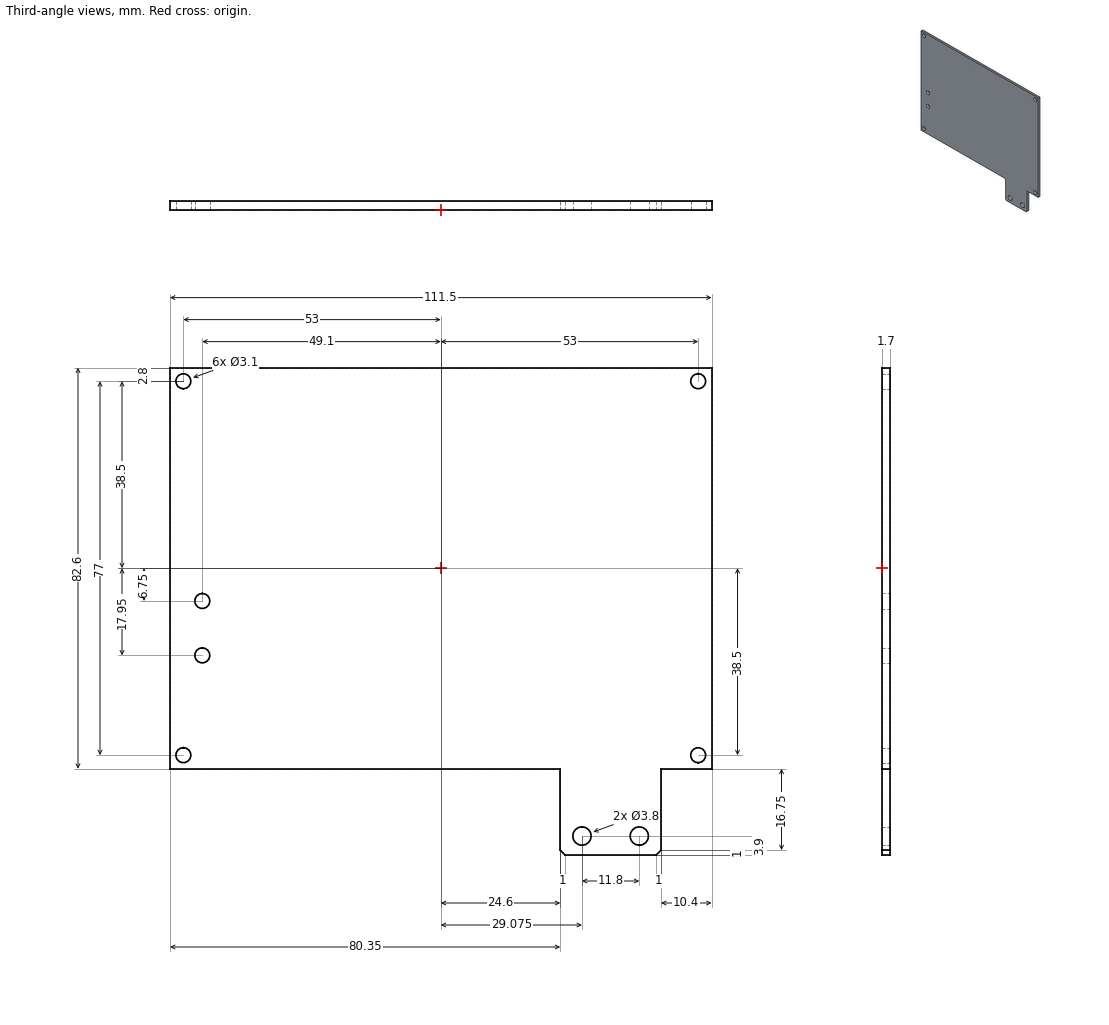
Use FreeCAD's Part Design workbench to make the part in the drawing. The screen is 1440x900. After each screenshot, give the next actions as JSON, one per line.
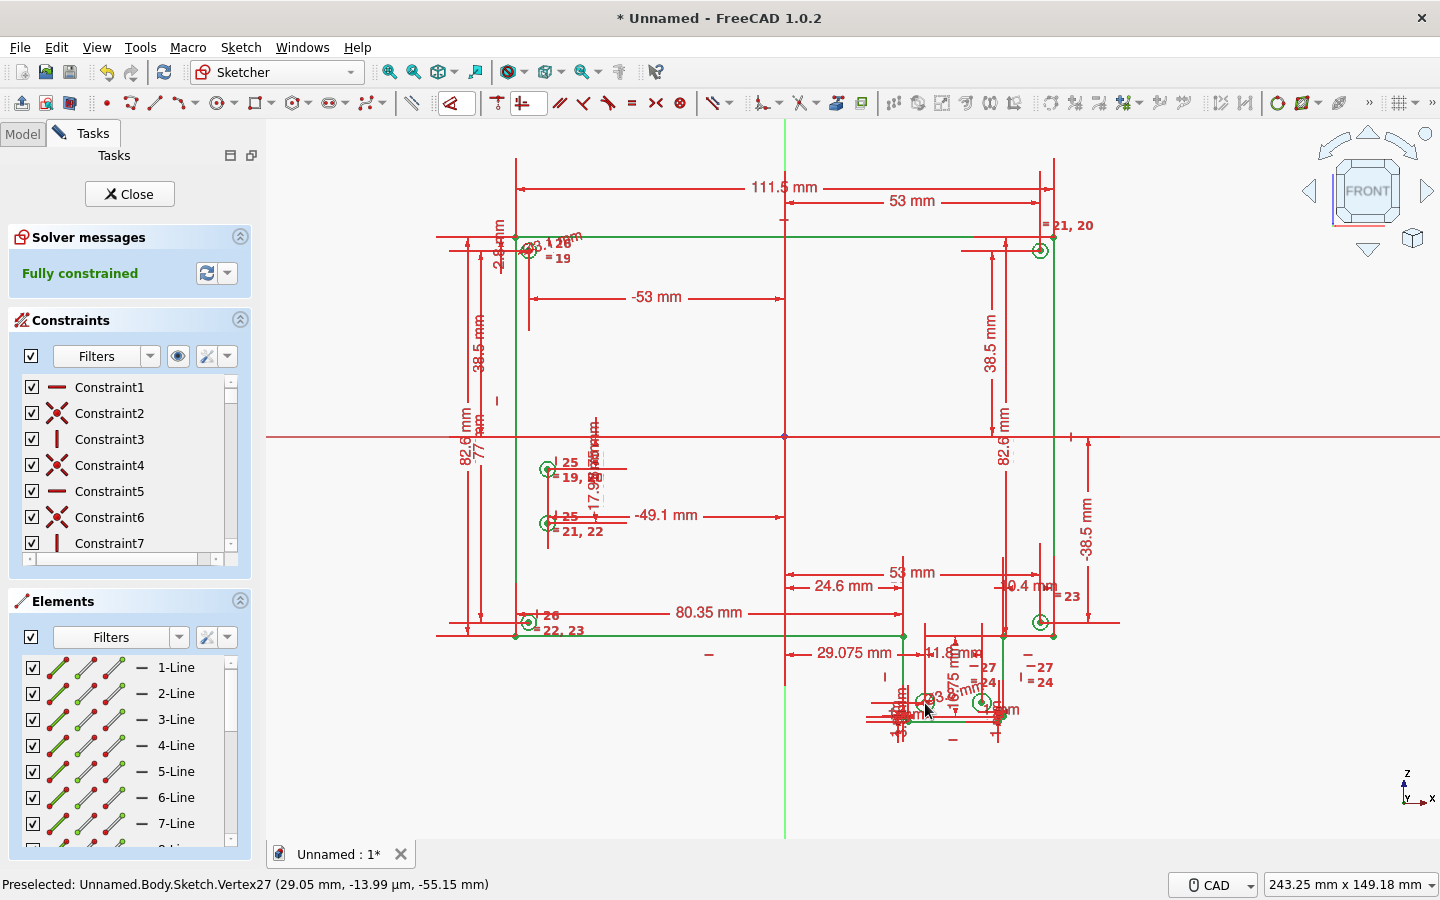
{"action": "left_click", "coordinate": [130, 194]}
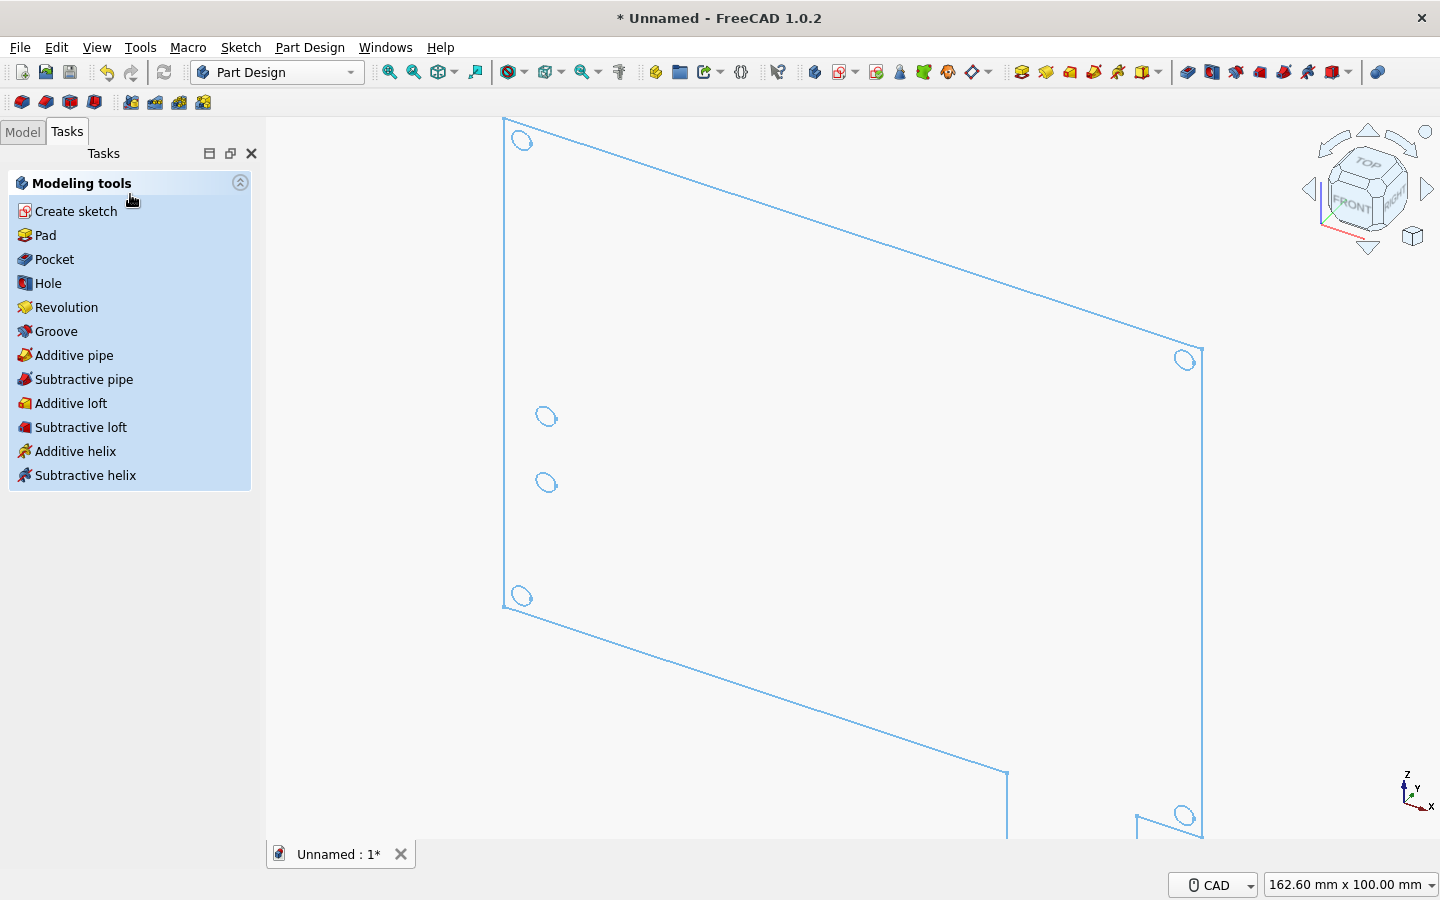
{"action": "left_click", "coordinate": [1022, 72]}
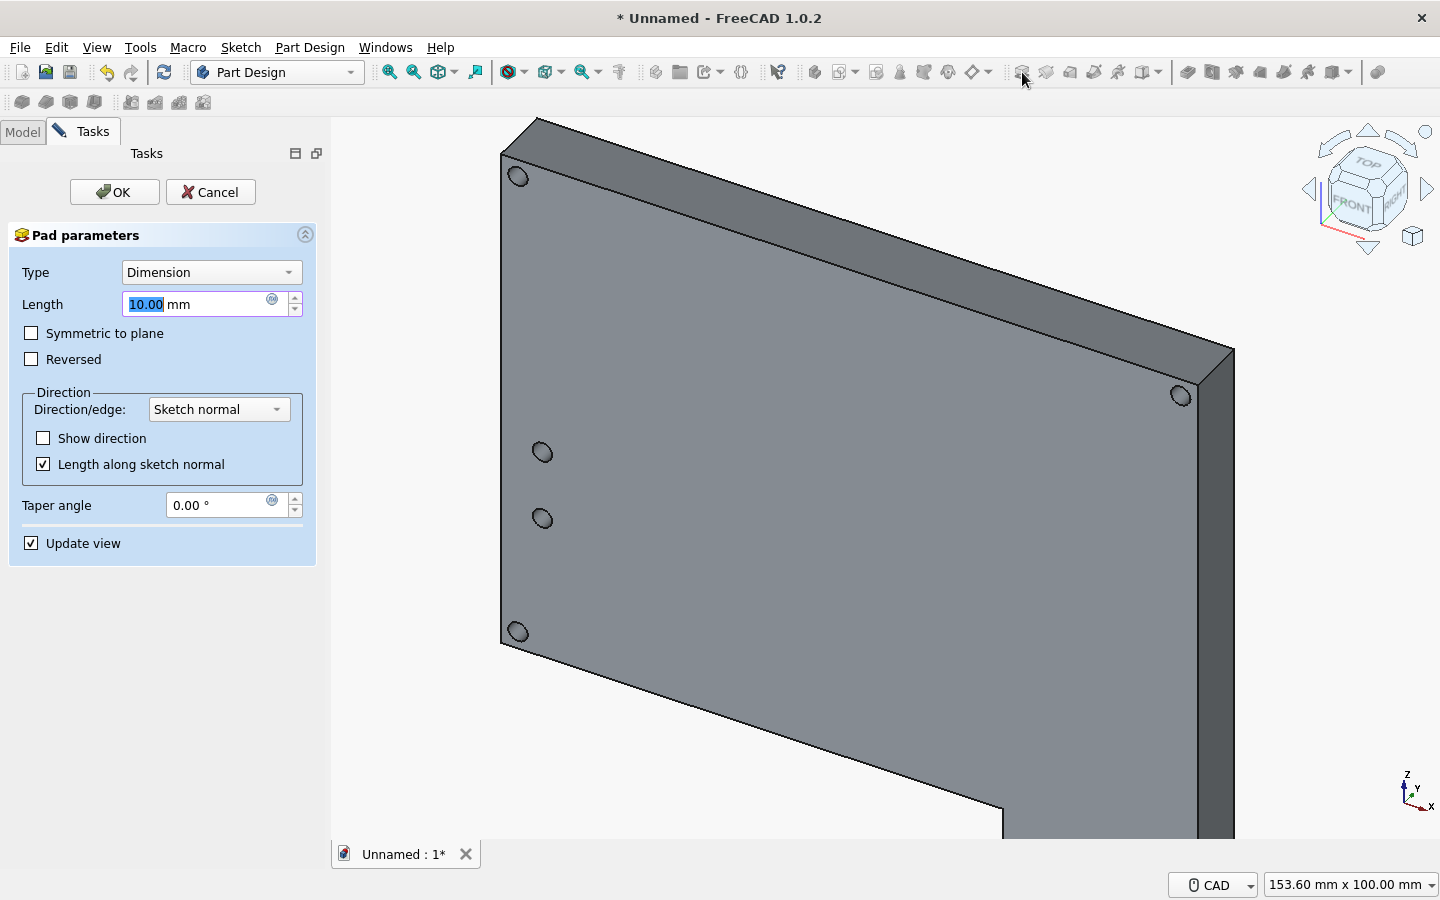
{"action": "type", "text": "1.7"}
{"action": "key", "text": "Tab"}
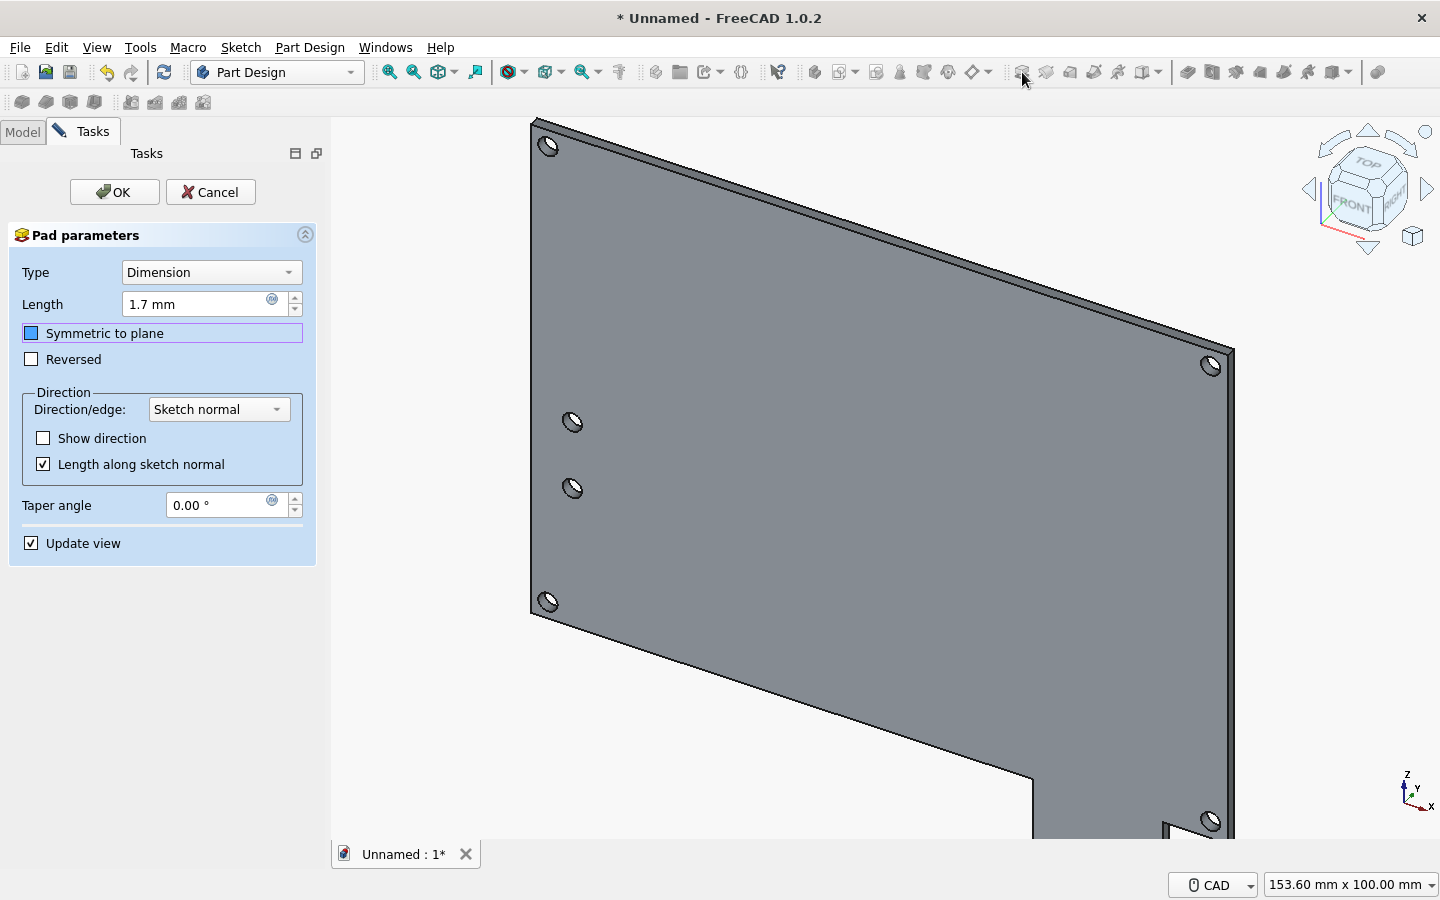
{"action": "left_click", "coordinate": [30, 359]}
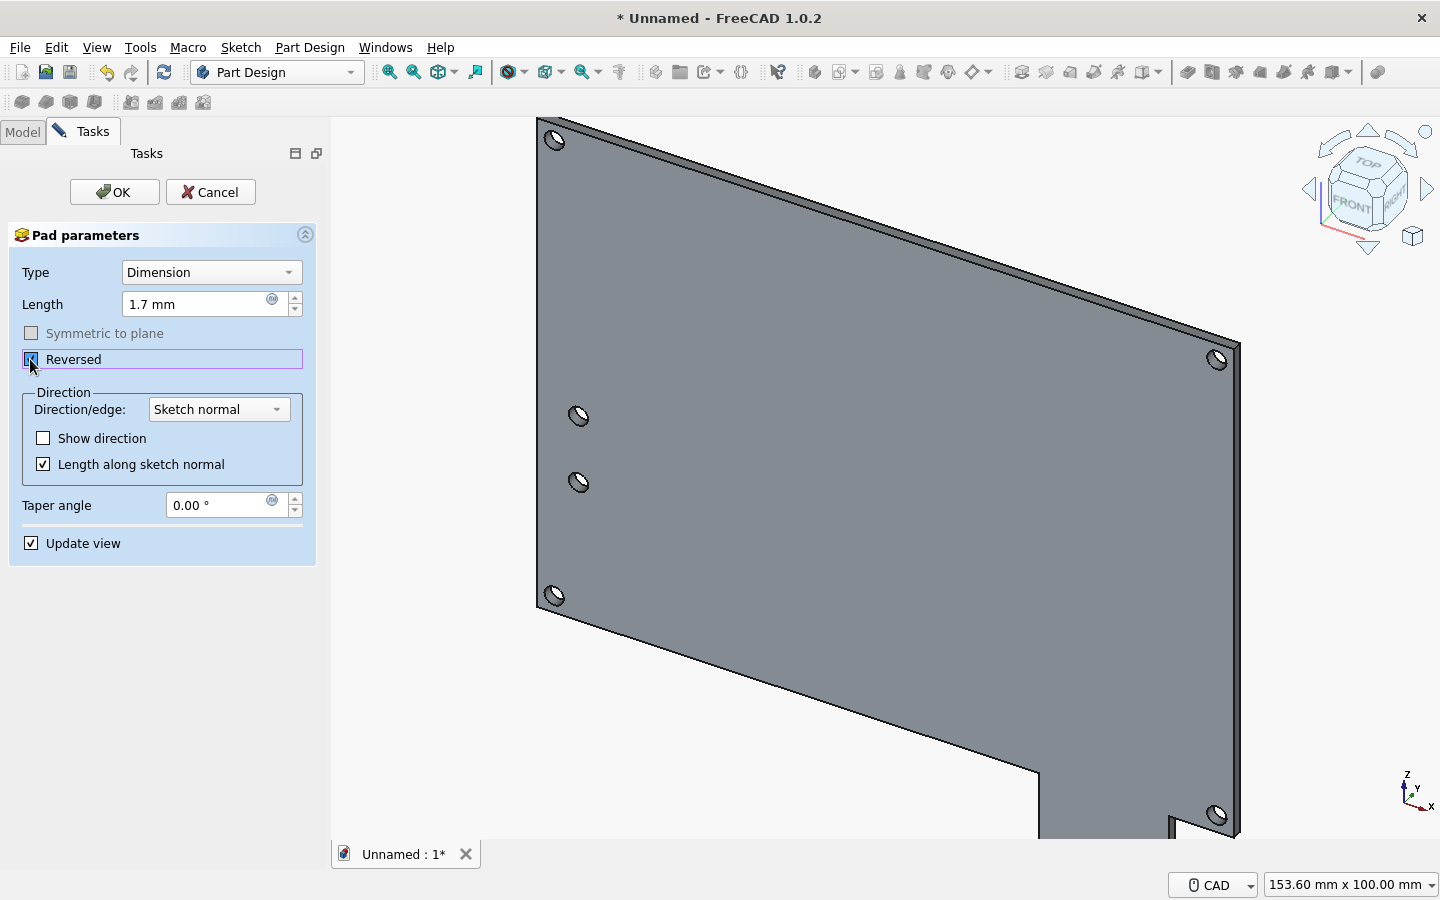
{"action": "left_click", "coordinate": [115, 192]}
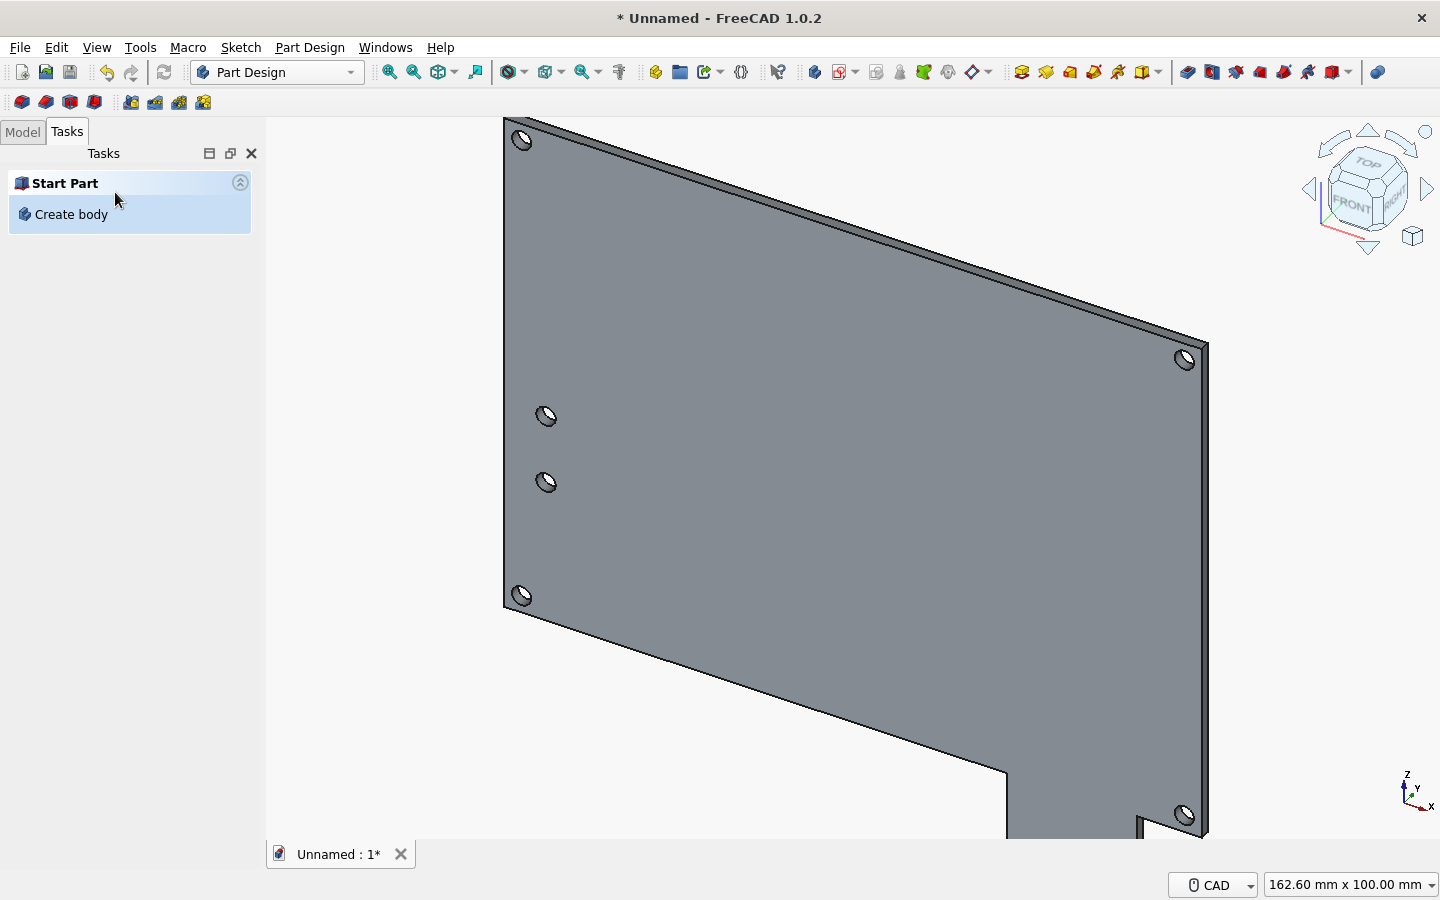
{"action": "key", "text": "0"}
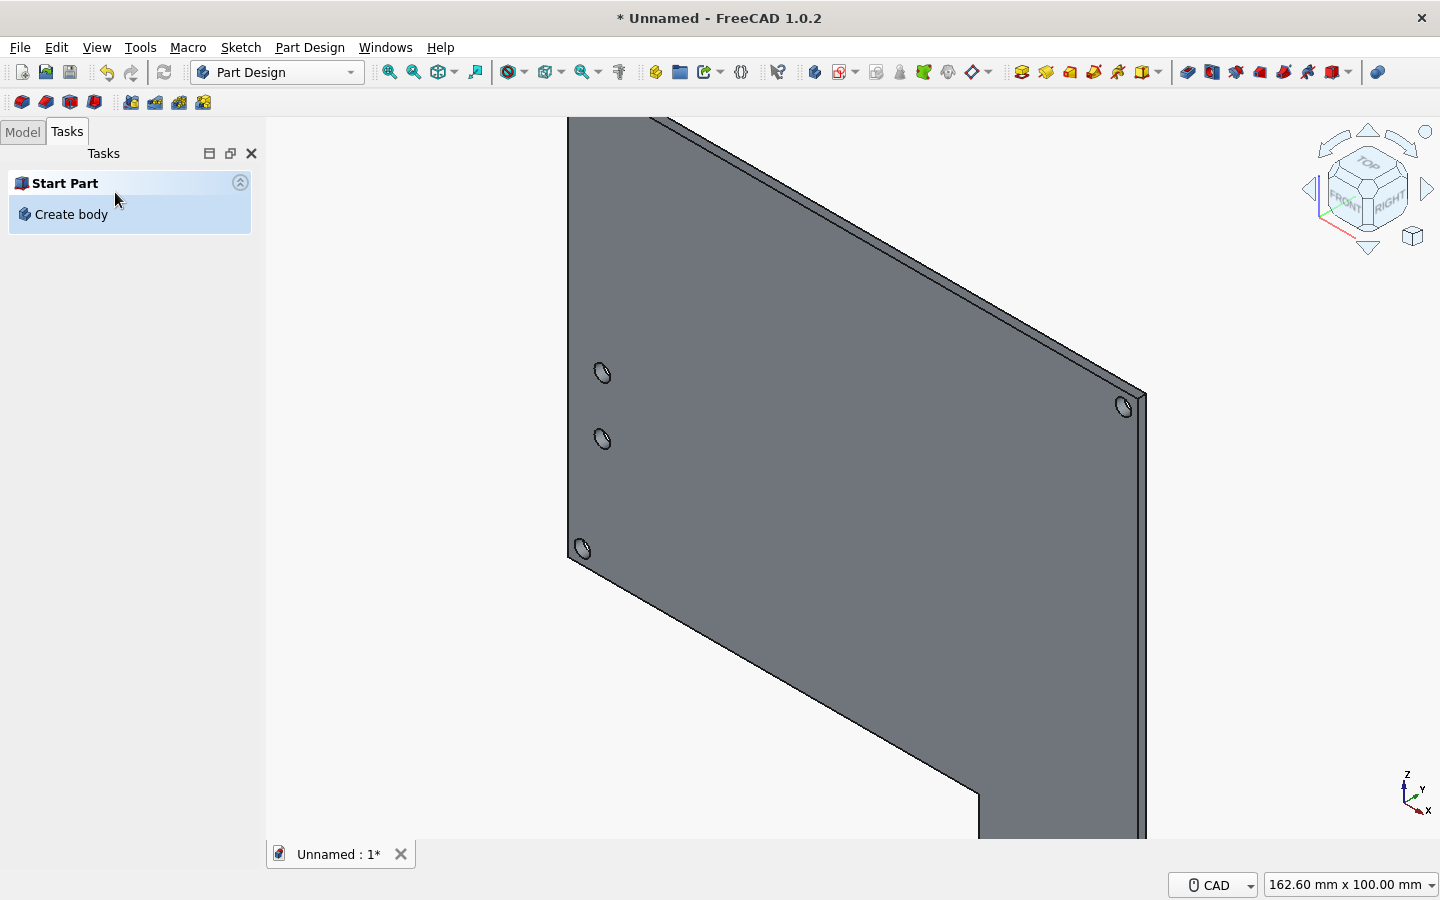
{"action": "left_click", "coordinate": [390, 72]}